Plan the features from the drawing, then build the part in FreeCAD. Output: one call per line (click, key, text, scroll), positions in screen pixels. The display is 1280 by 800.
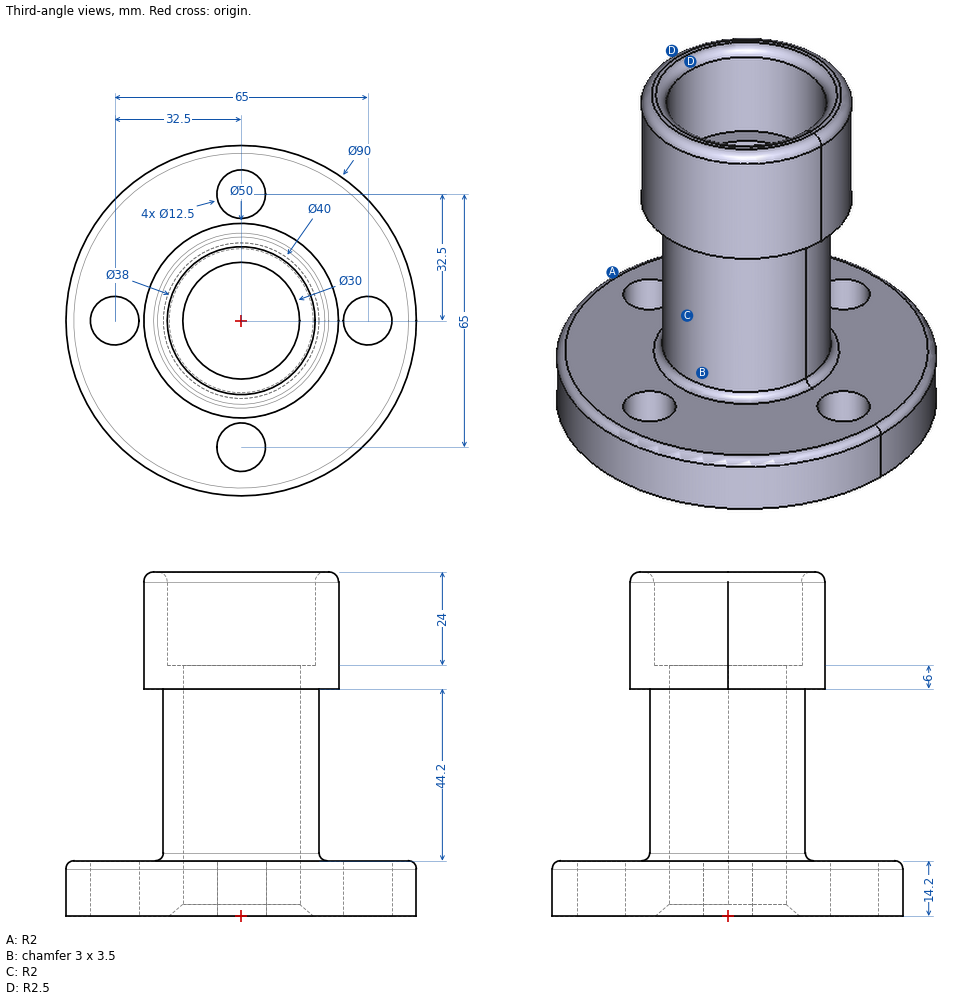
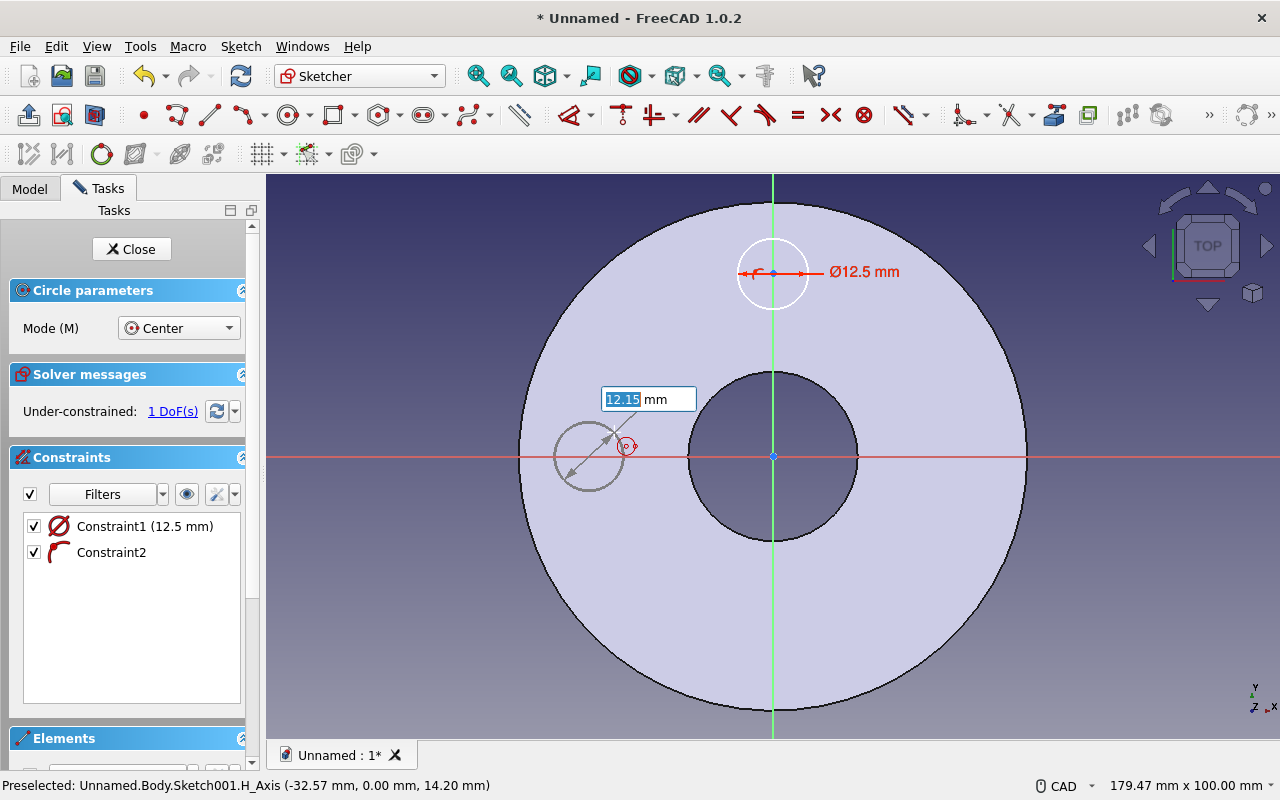
text(12.5)
key(Return)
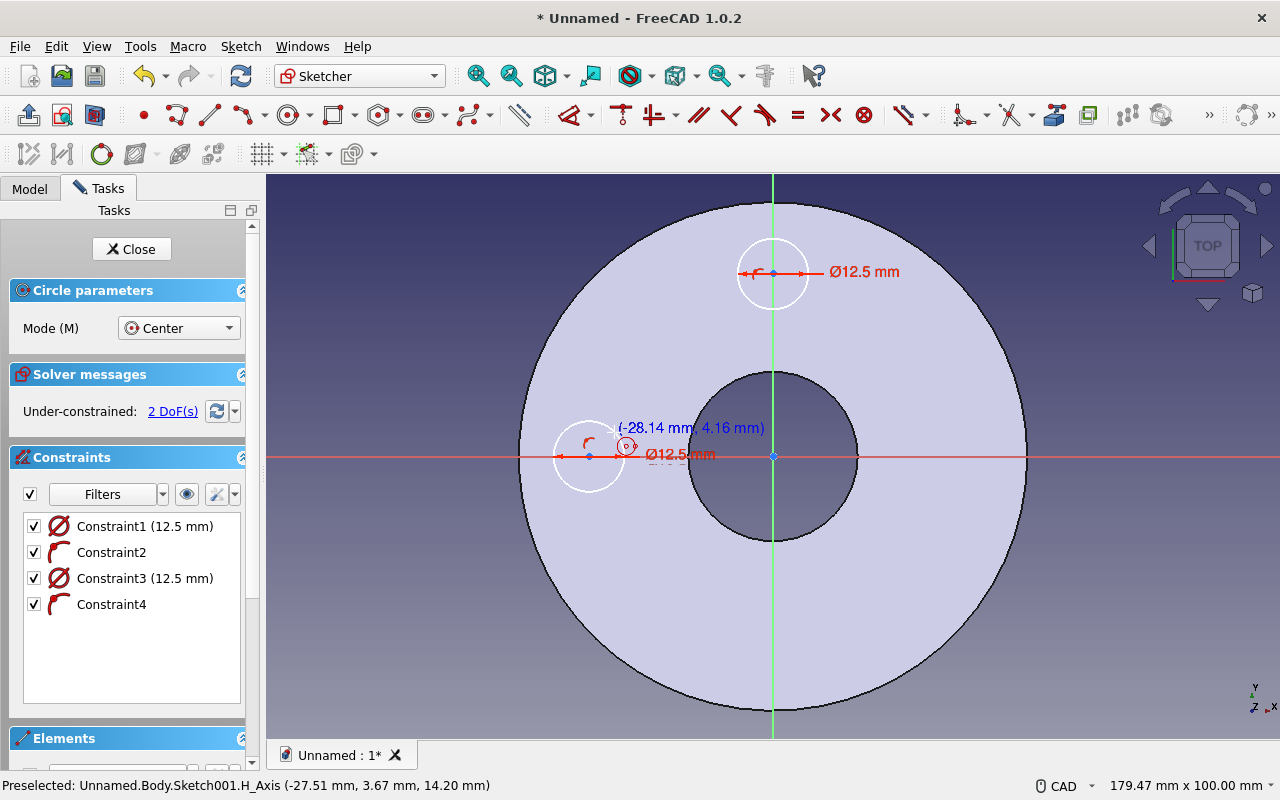
click(957, 456)
move(982, 432)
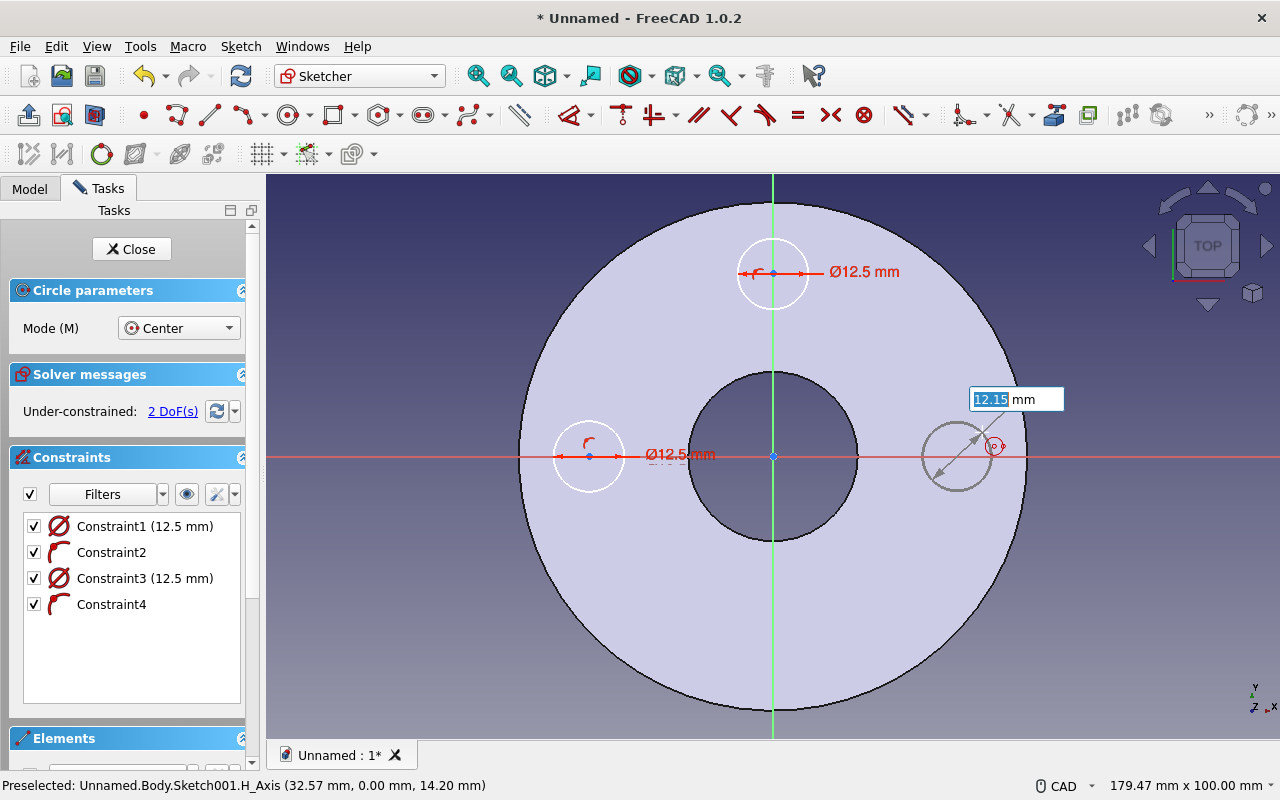
text(12.5)
key(Return)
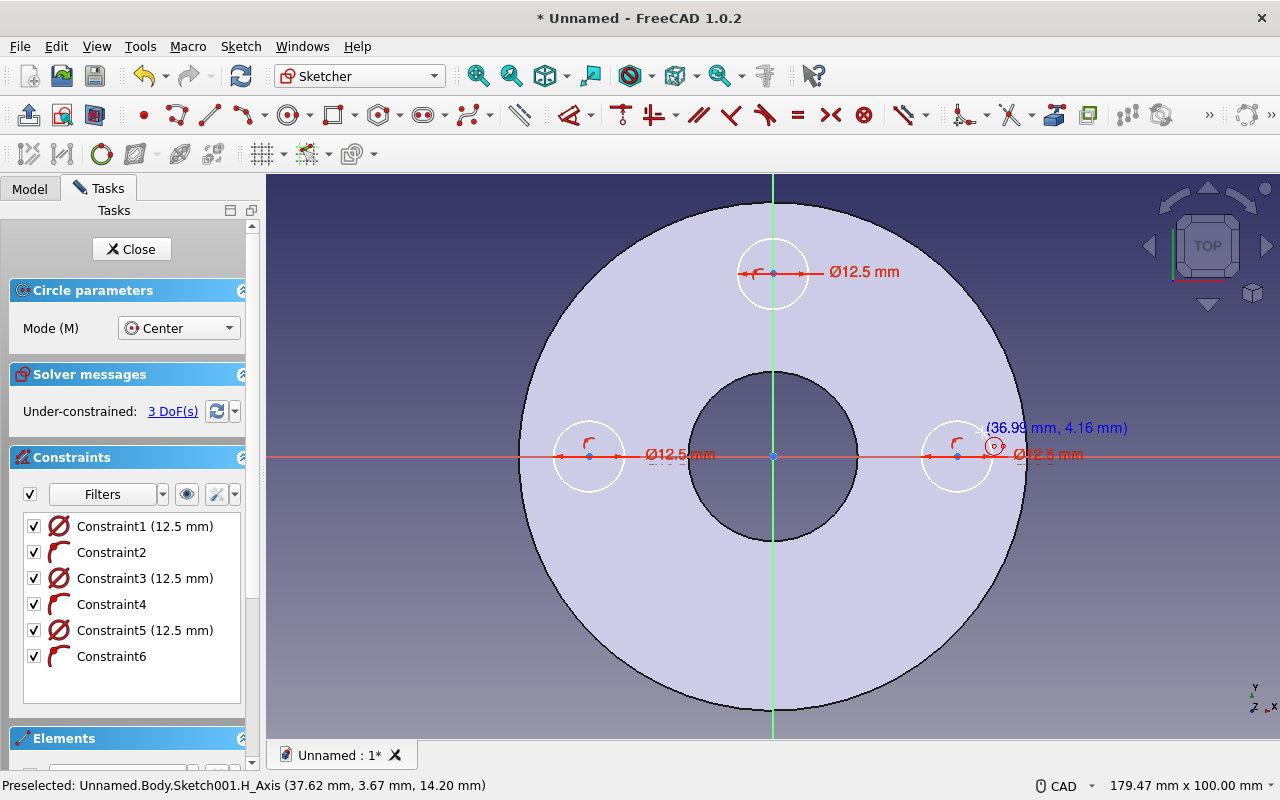
click(773, 640)
move(798, 615)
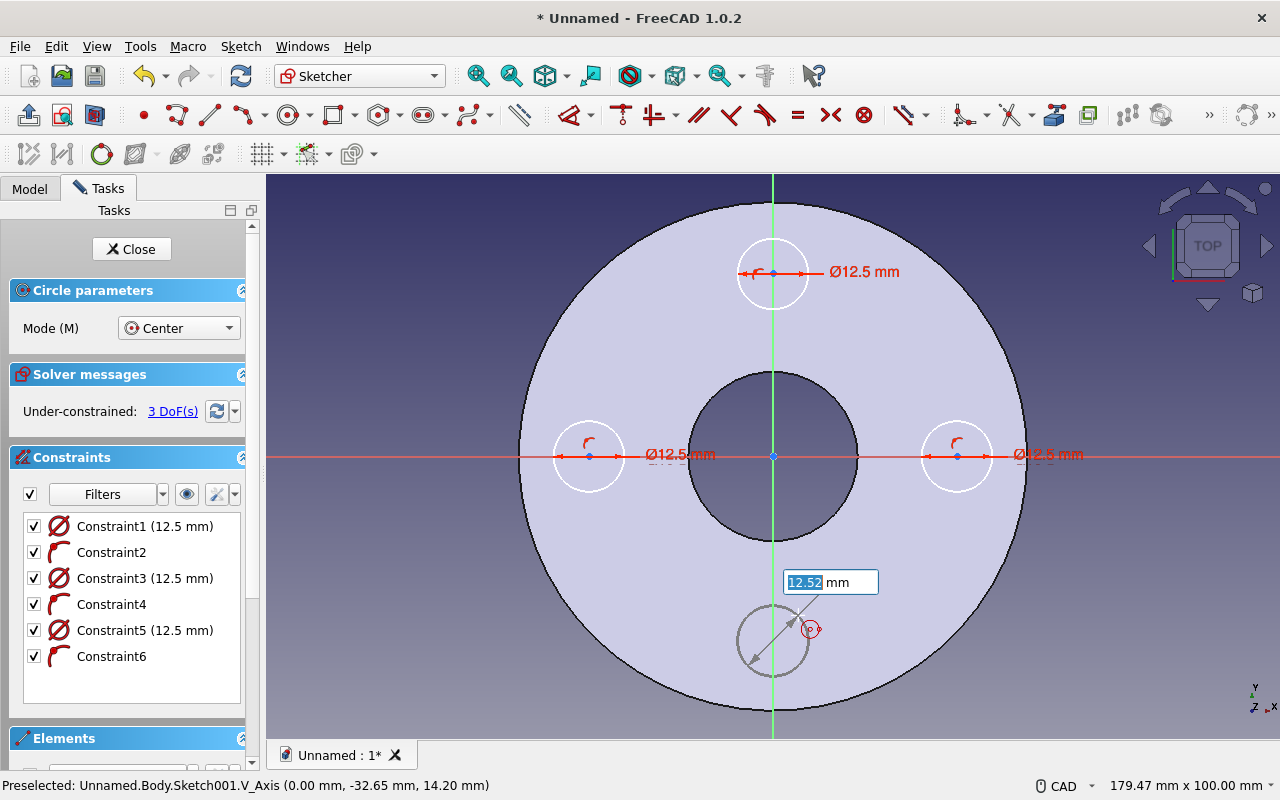
text(12.5)
key(Return)
key(Escape)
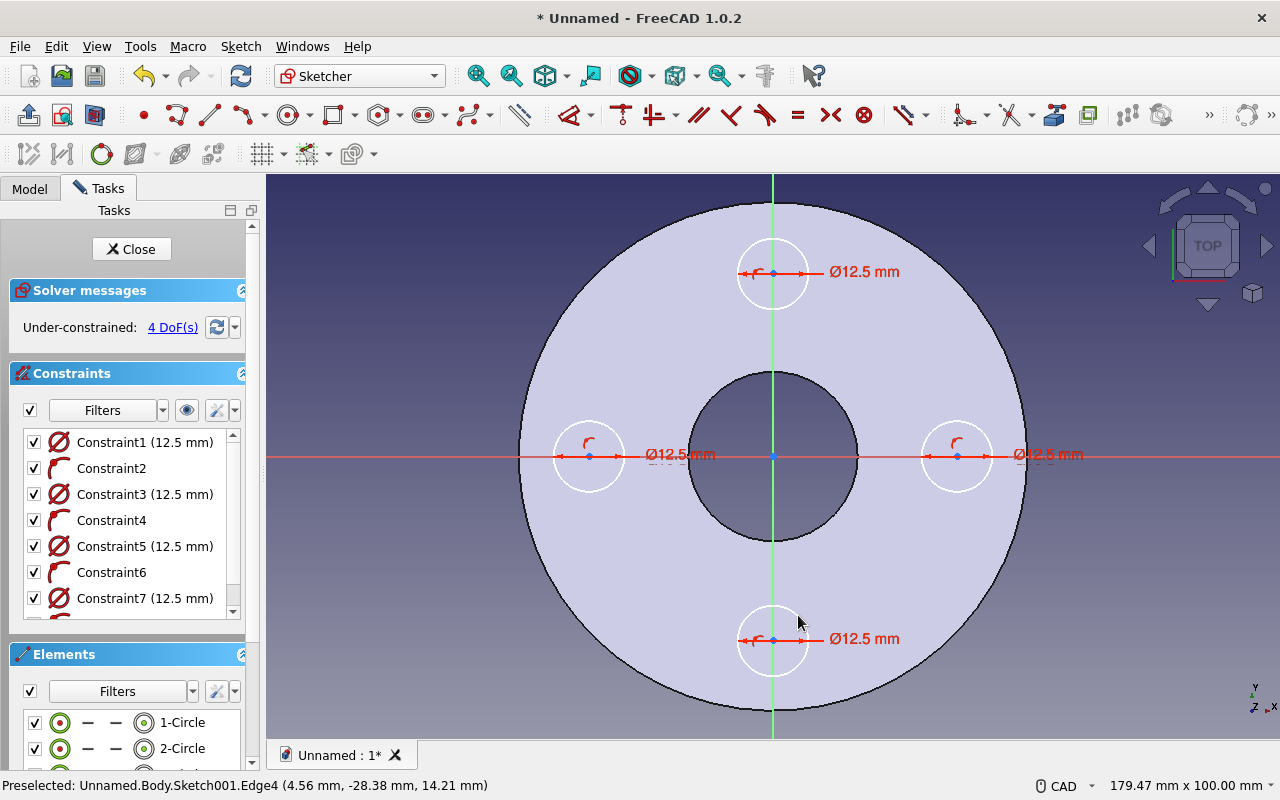
click(568, 116)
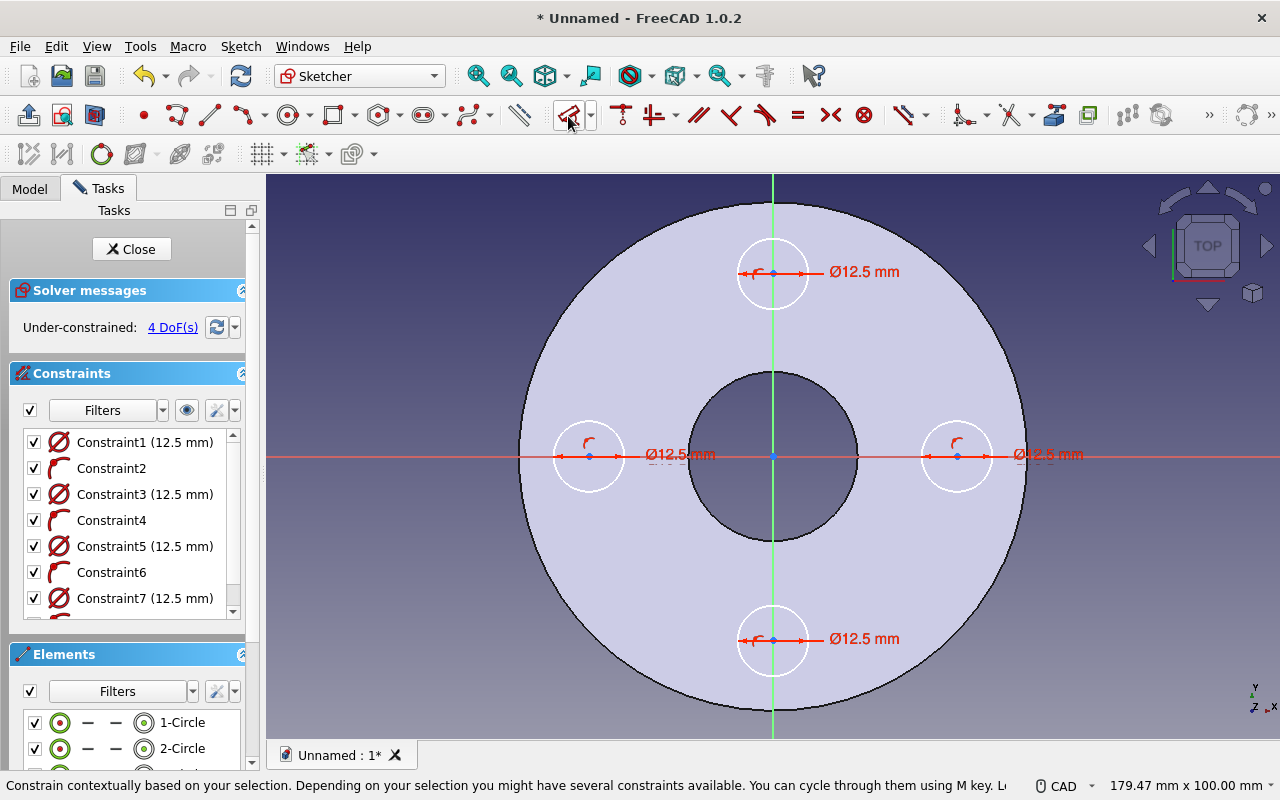
click(589, 456)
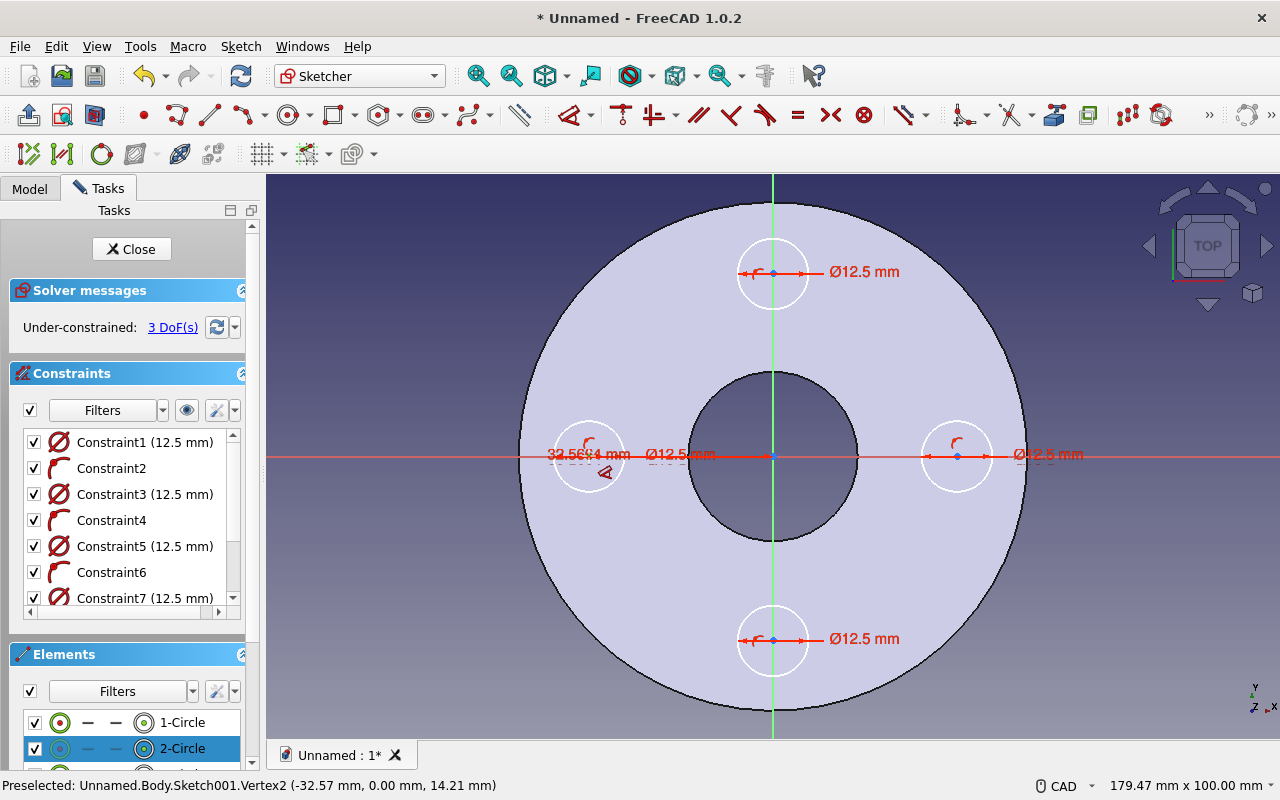
click(957, 456)
click(688, 490)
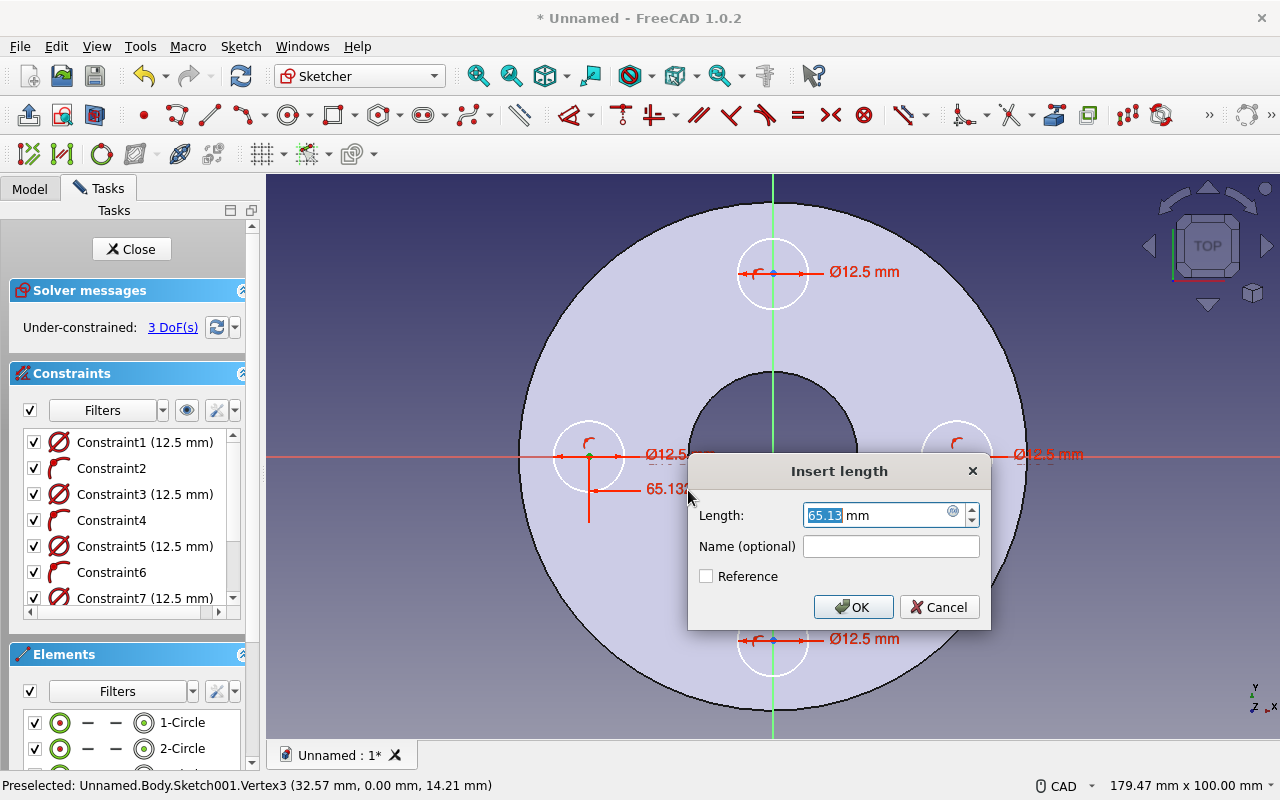
text(65)
key(Return)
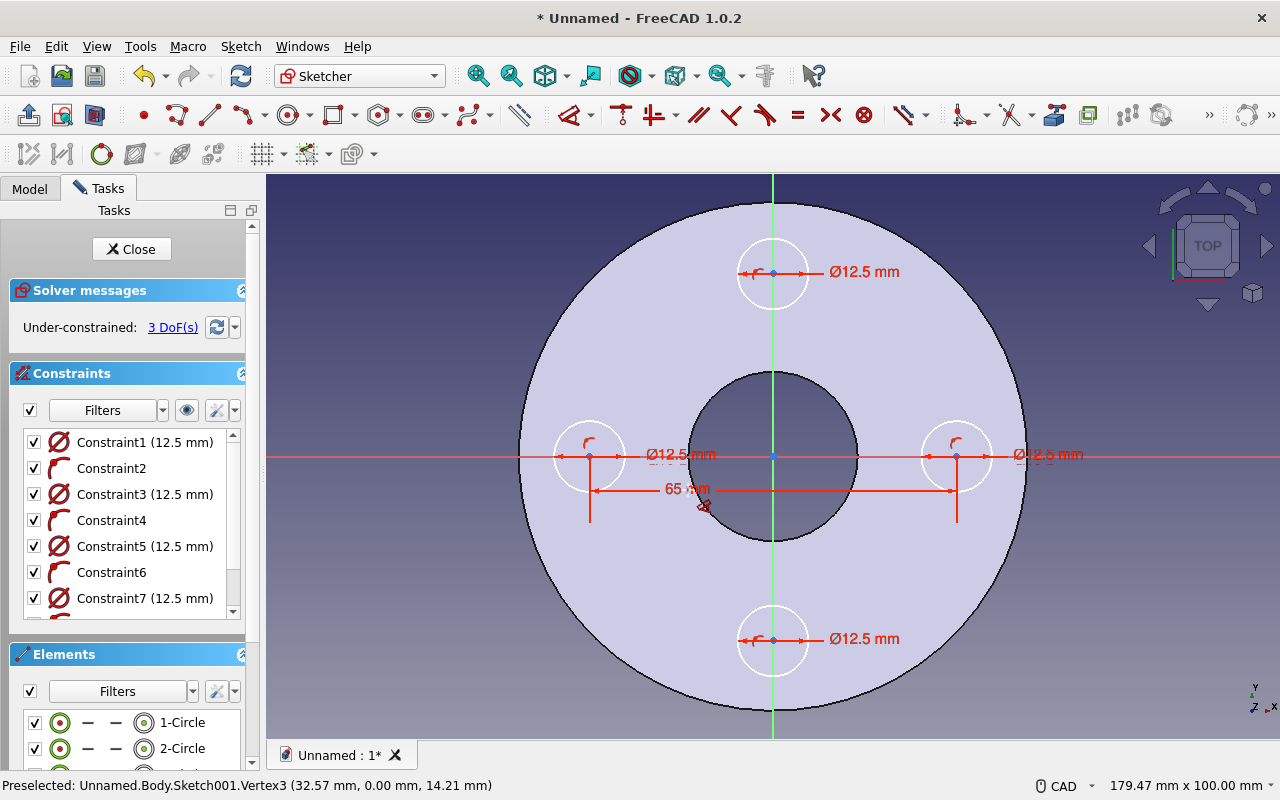
click(773, 274)